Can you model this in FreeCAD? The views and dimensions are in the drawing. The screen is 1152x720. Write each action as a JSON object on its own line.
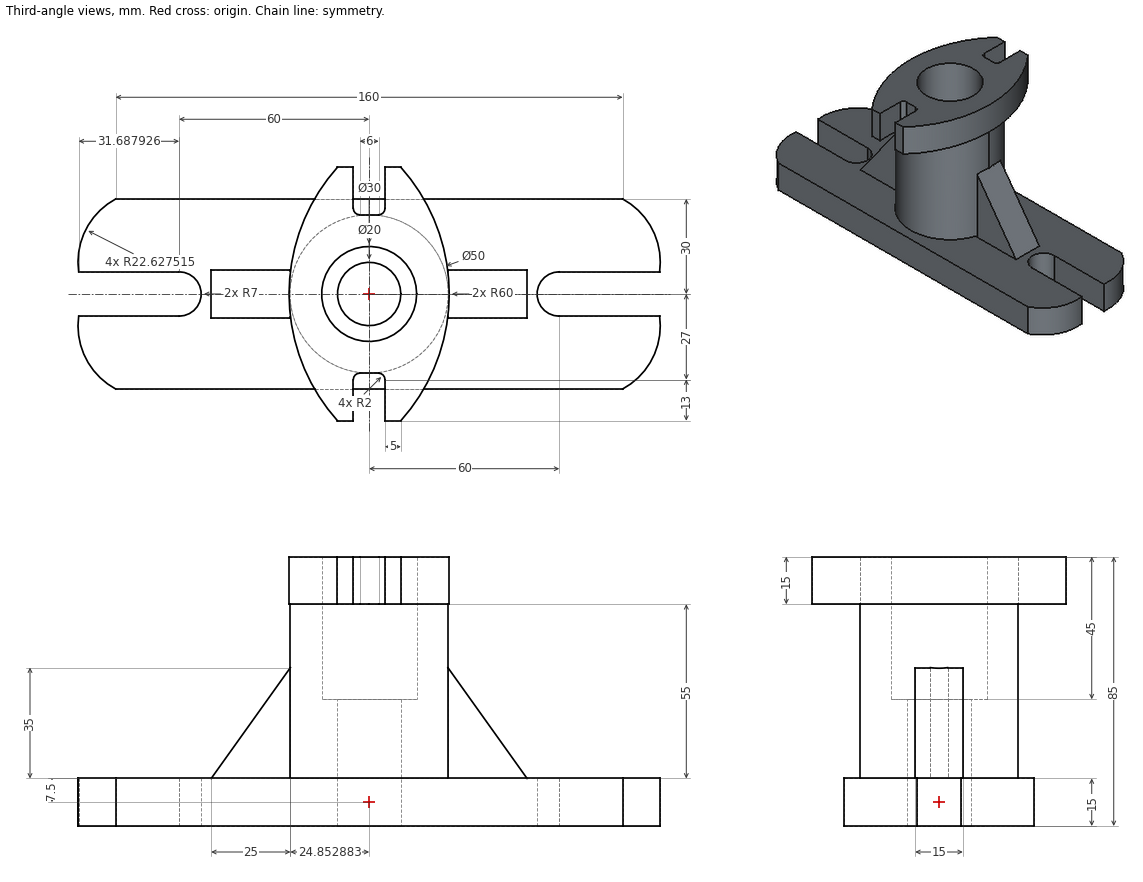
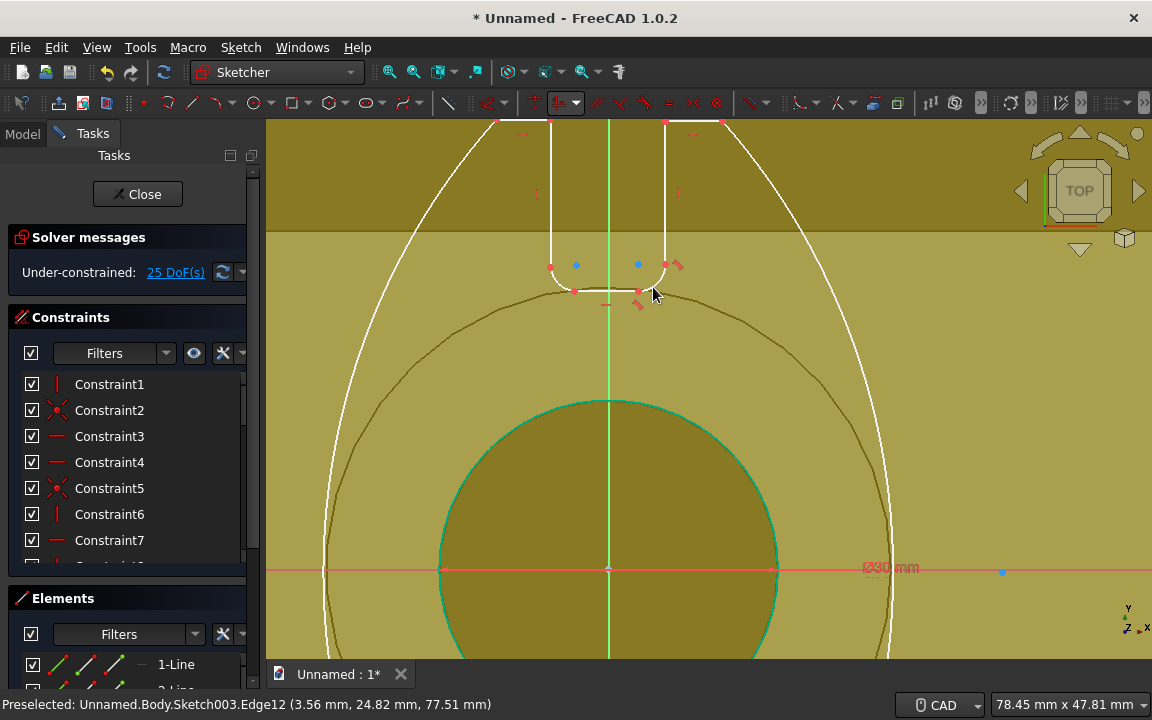
{"action": "scroll", "coordinate": [620, 291], "scroll_direction": "up", "scroll_amount": 2}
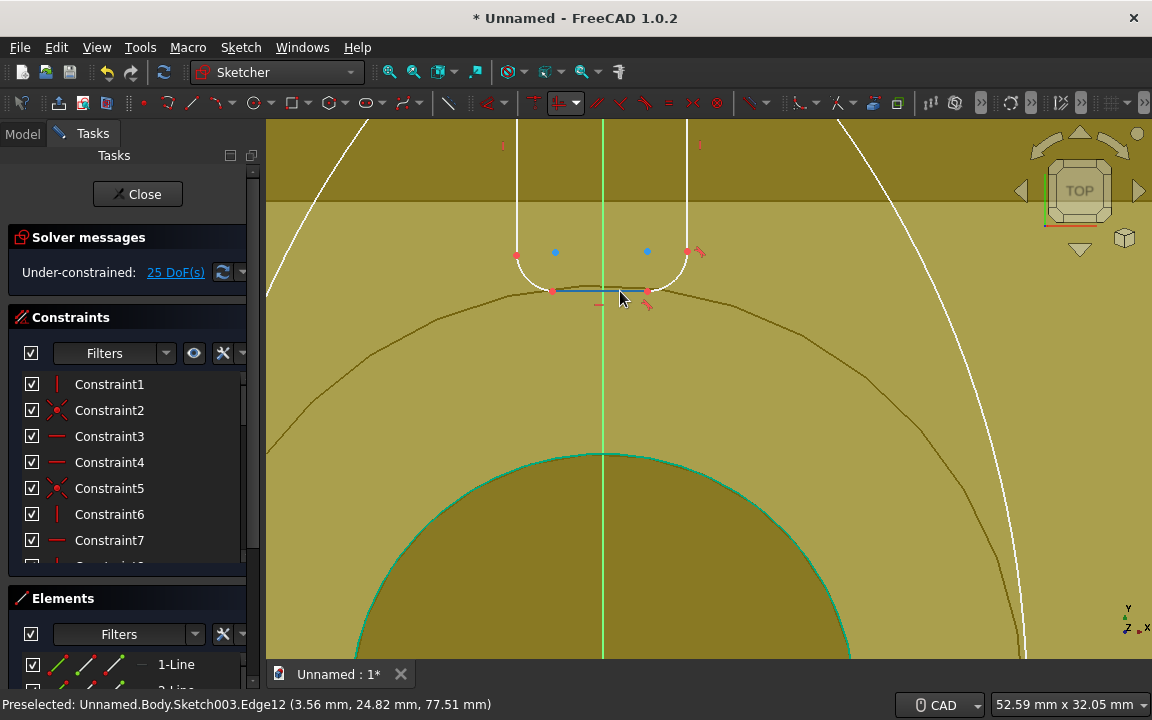
{"action": "left_click", "coordinate": [619, 291]}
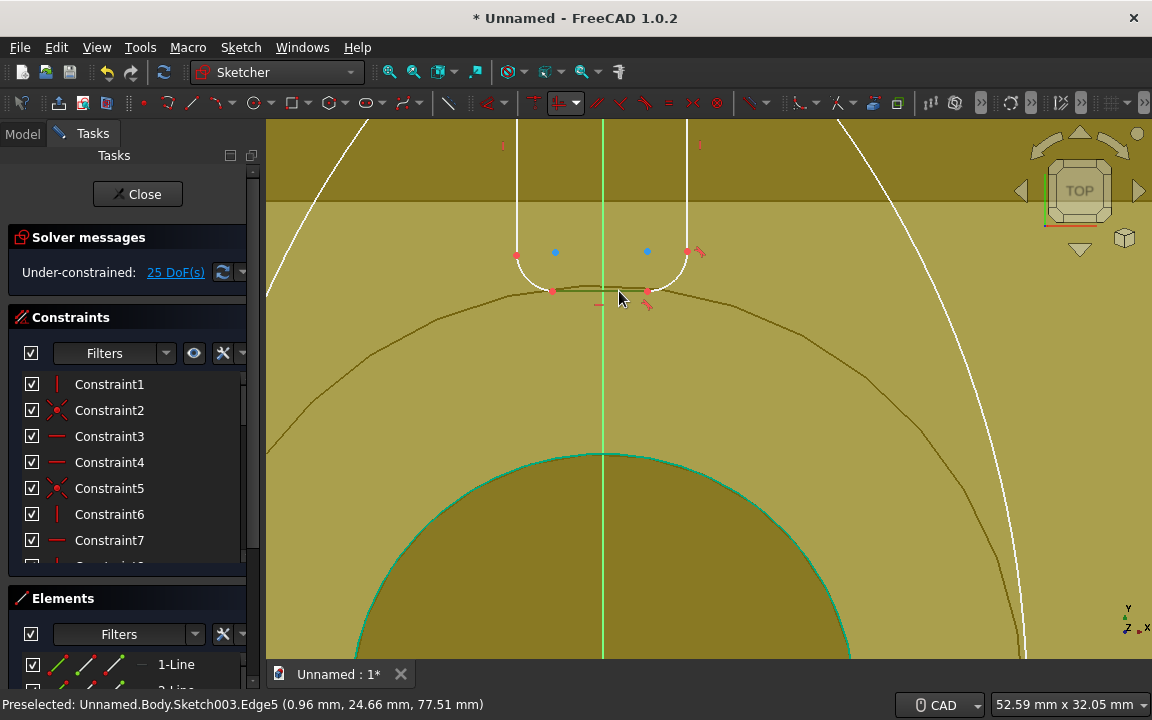
{"action": "left_click", "coordinate": [521, 271]}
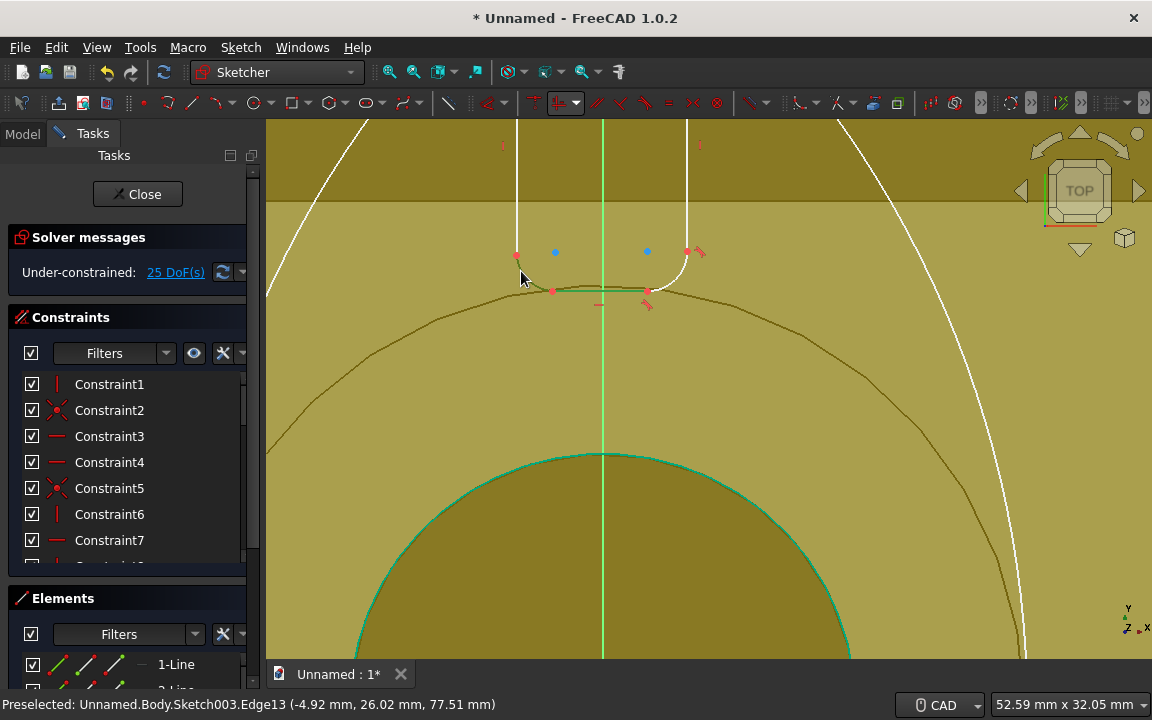
{"action": "left_click", "coordinate": [646, 104]}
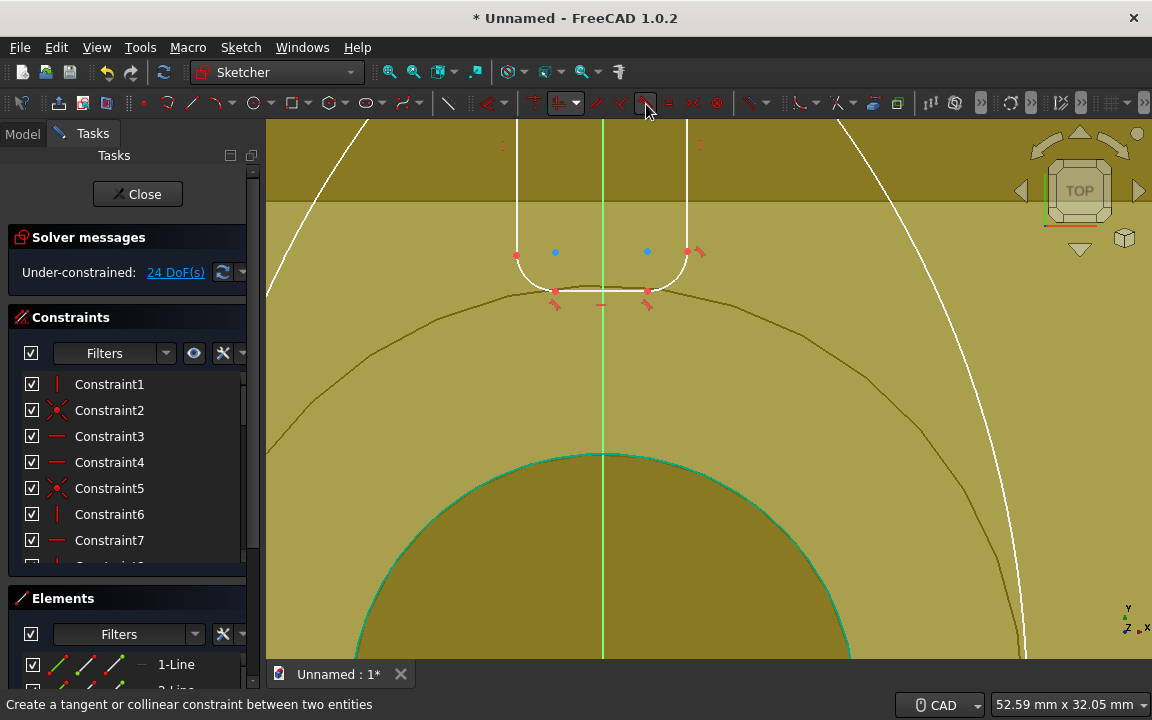
{"action": "scroll", "coordinate": [653, 285], "scroll_direction": "down", "scroll_amount": 7}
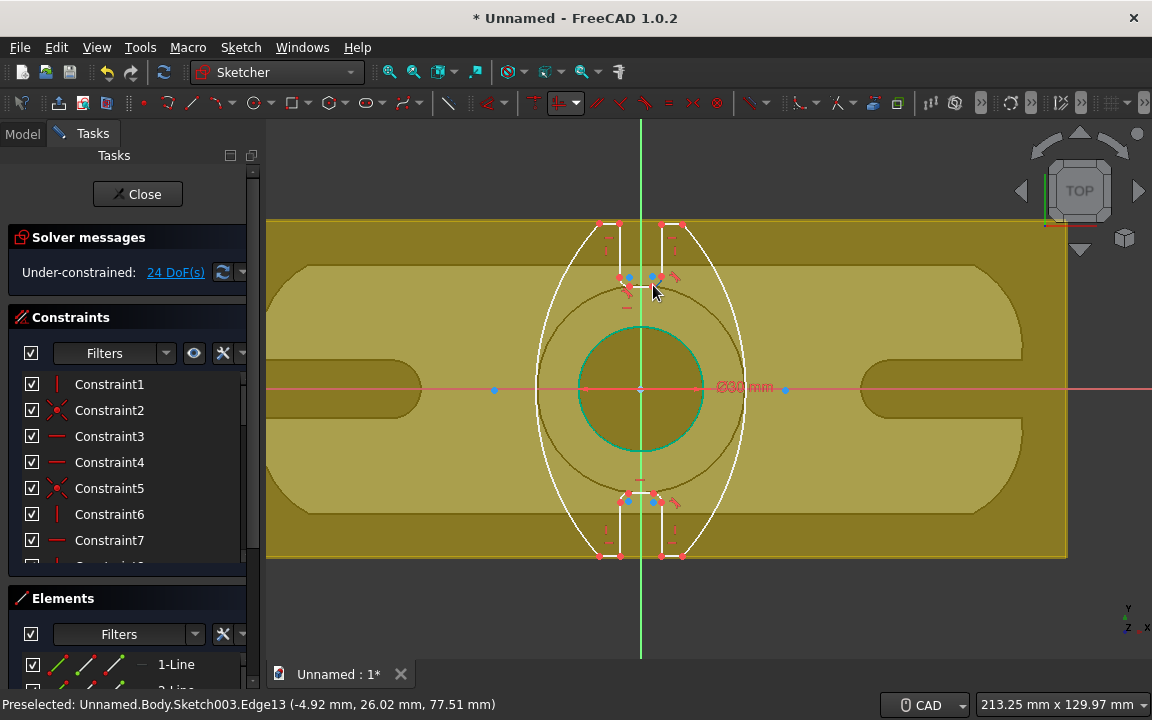
{"action": "left_click", "coordinate": [620, 262]}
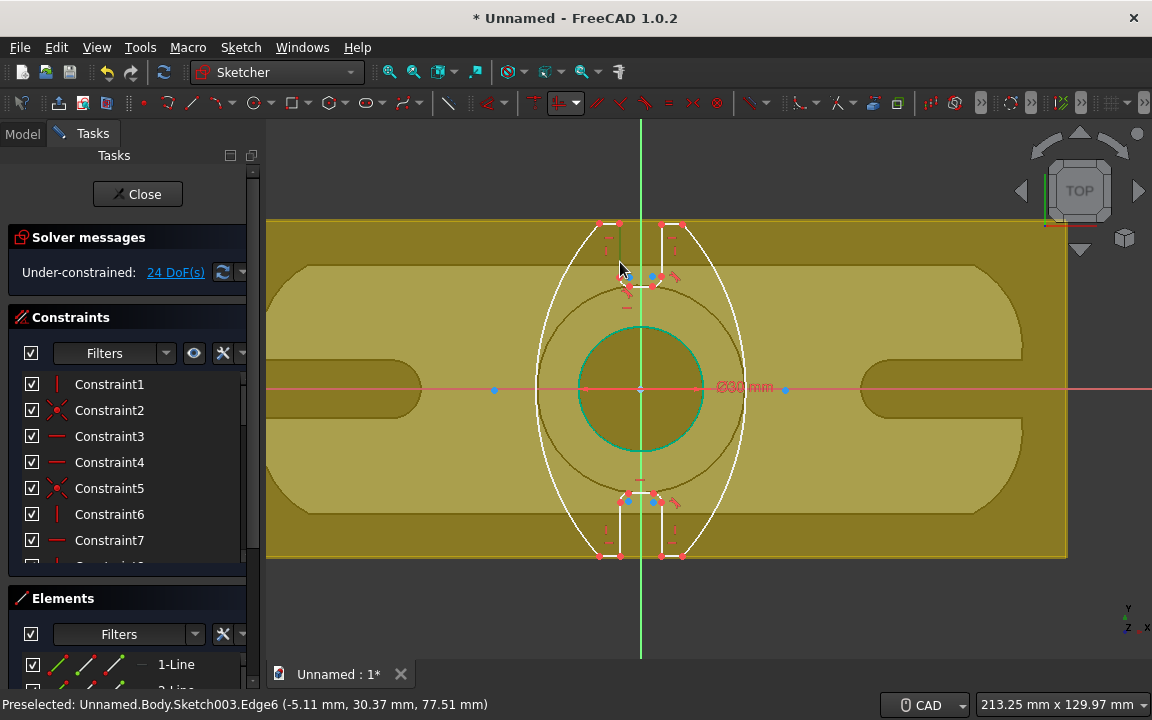
{"action": "scroll", "coordinate": [623, 284], "scroll_direction": "up", "scroll_amount": 4}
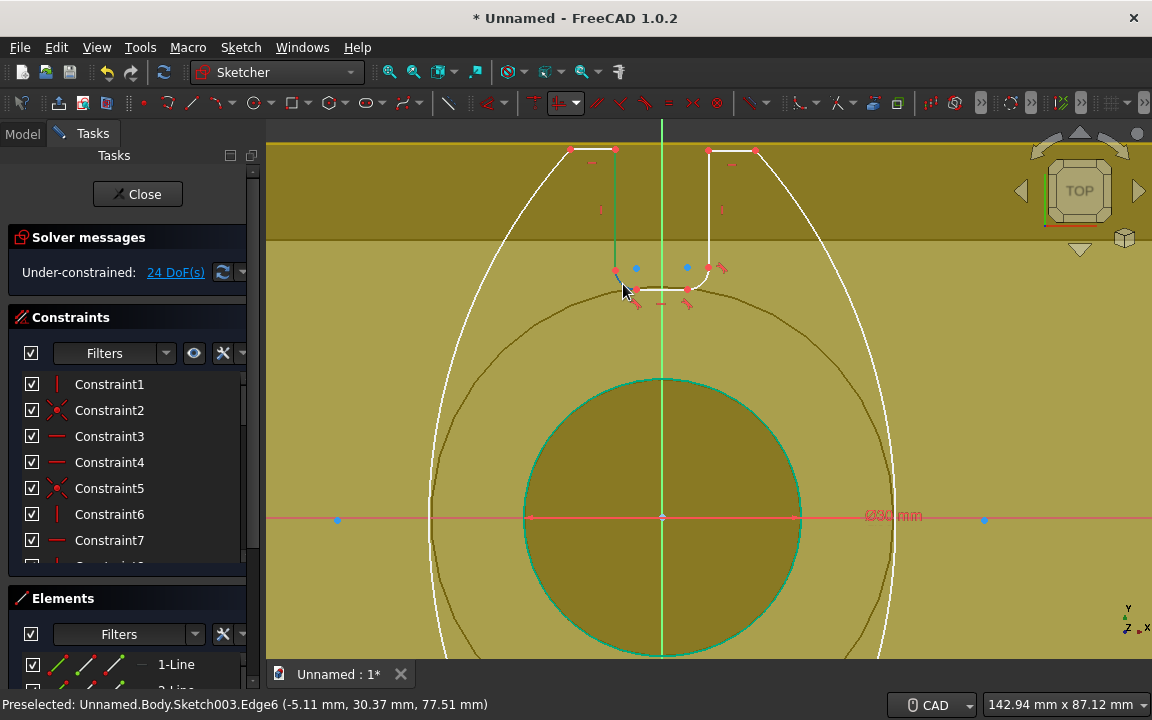
{"action": "left_click", "coordinate": [622, 284]}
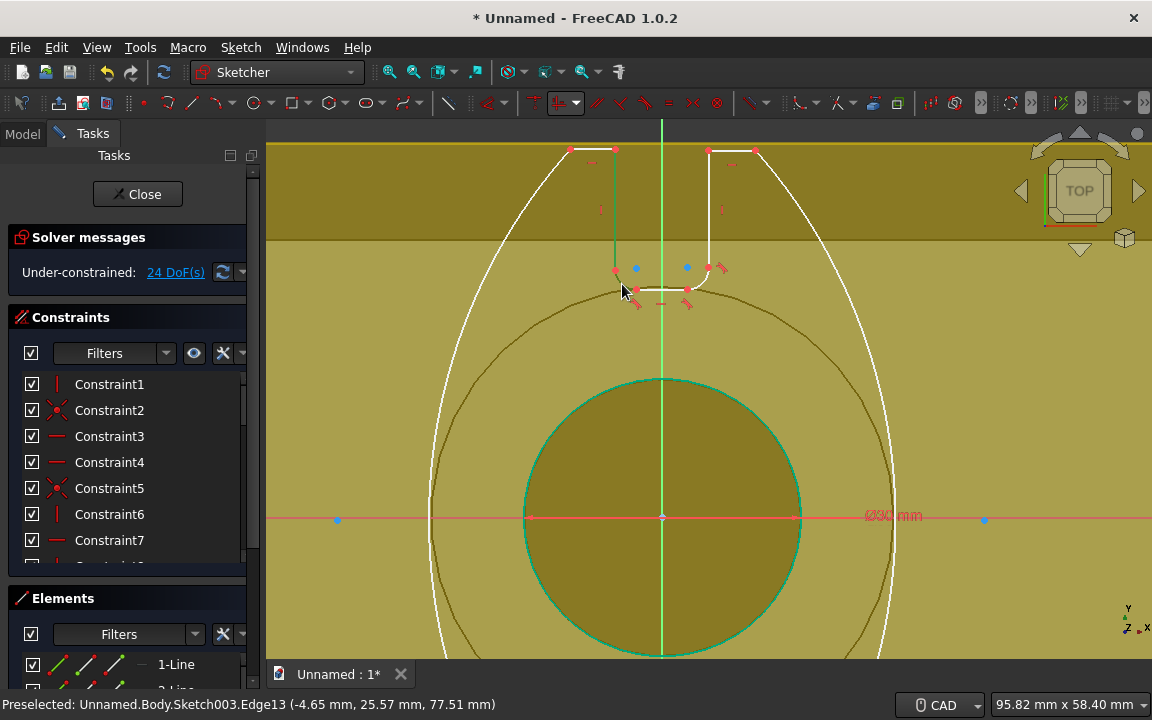
{"action": "key", "text": "t"}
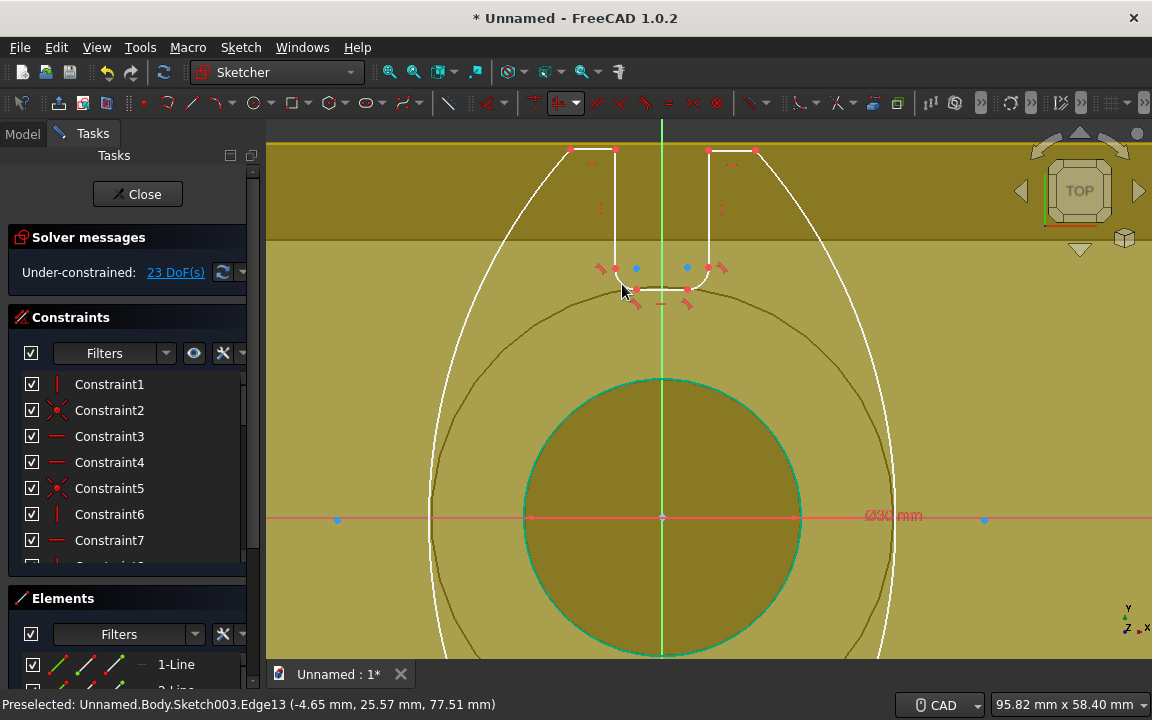
{"action": "scroll", "coordinate": [623, 284], "scroll_direction": "down", "scroll_amount": 4}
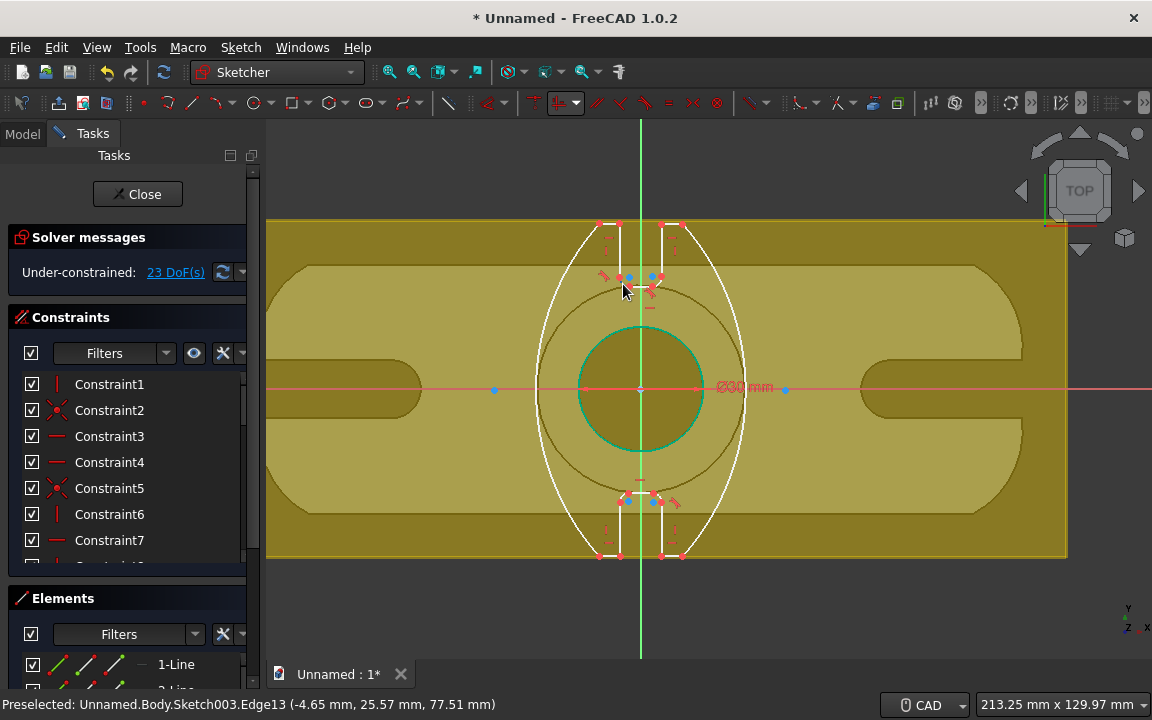
{"action": "left_click", "coordinate": [620, 540]}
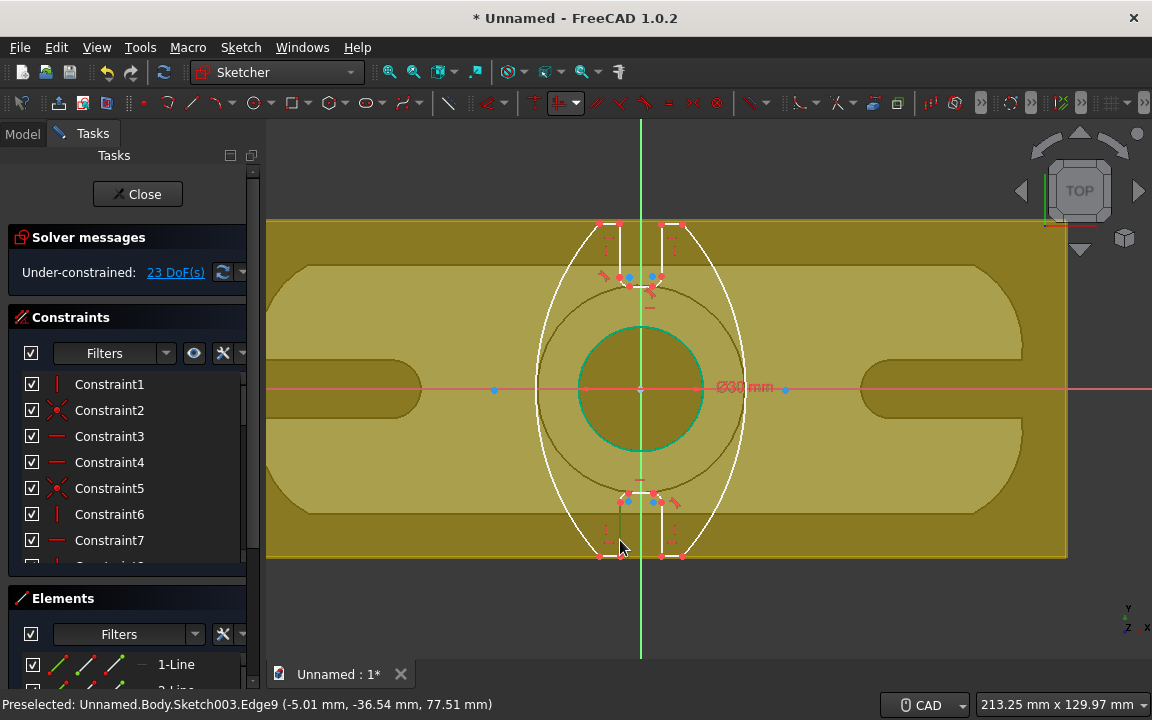
{"action": "scroll", "coordinate": [622, 496], "scroll_direction": "up", "scroll_amount": 4}